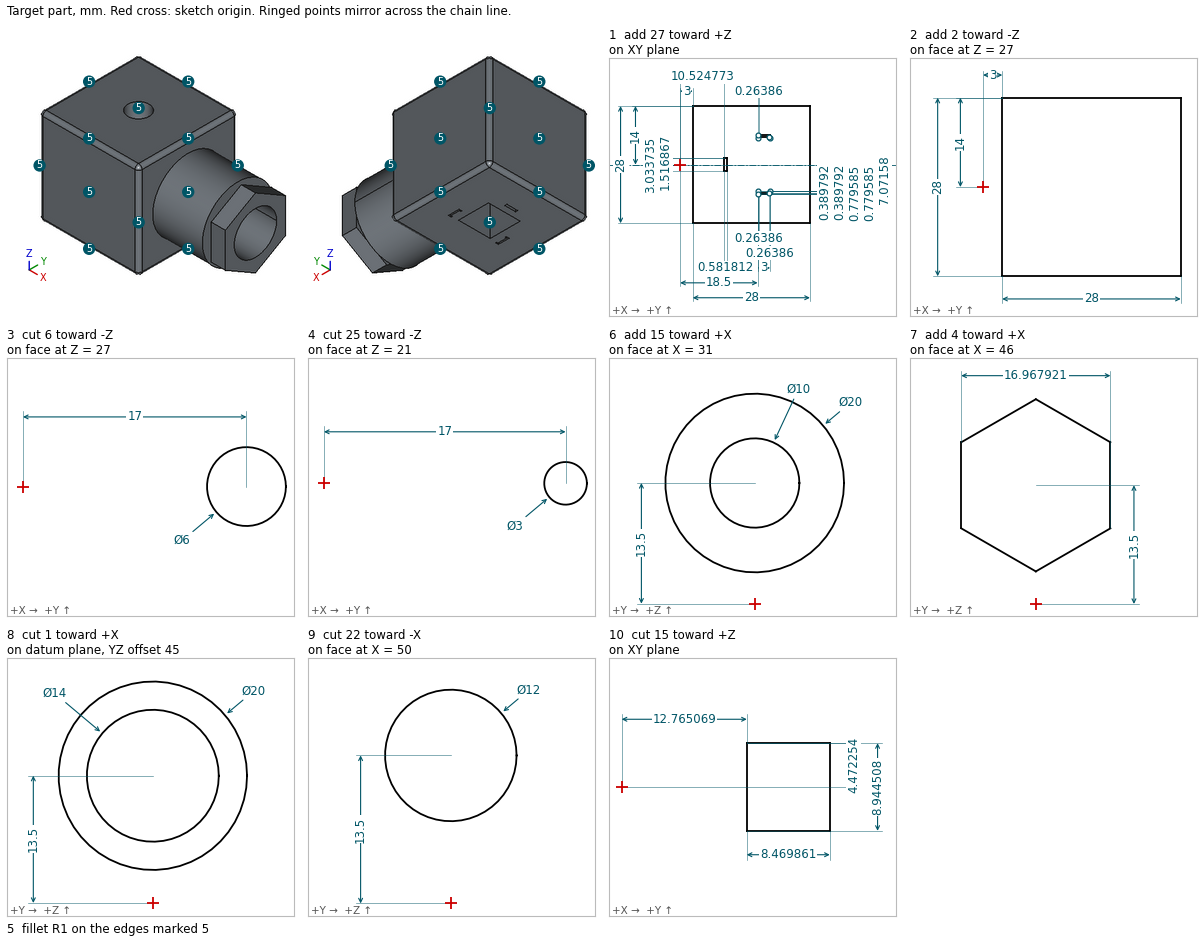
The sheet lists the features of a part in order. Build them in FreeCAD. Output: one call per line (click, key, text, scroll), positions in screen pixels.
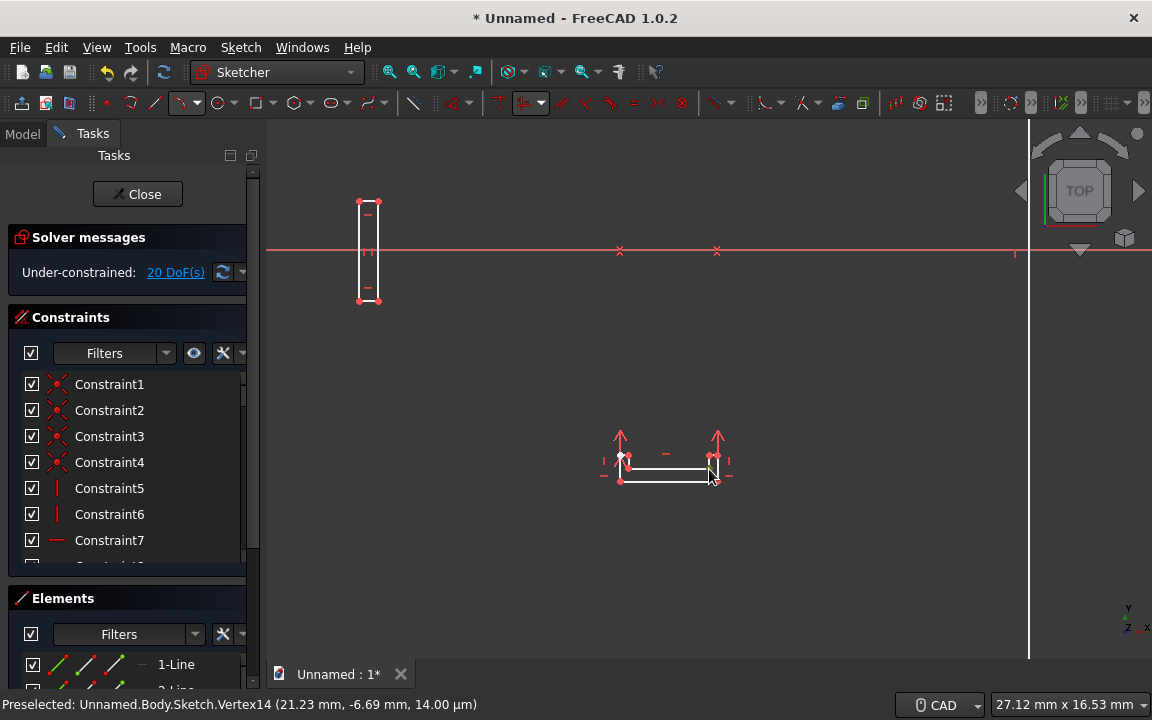
scroll(709, 470, down, 5)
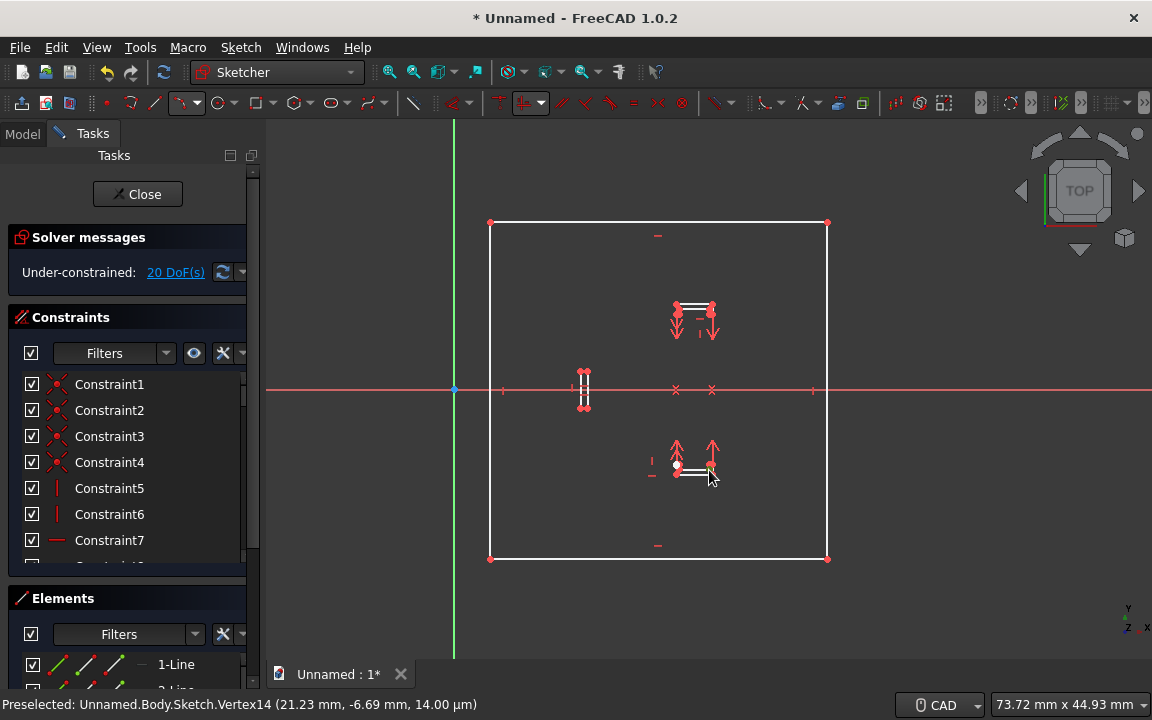
scroll(709, 309, up, 5)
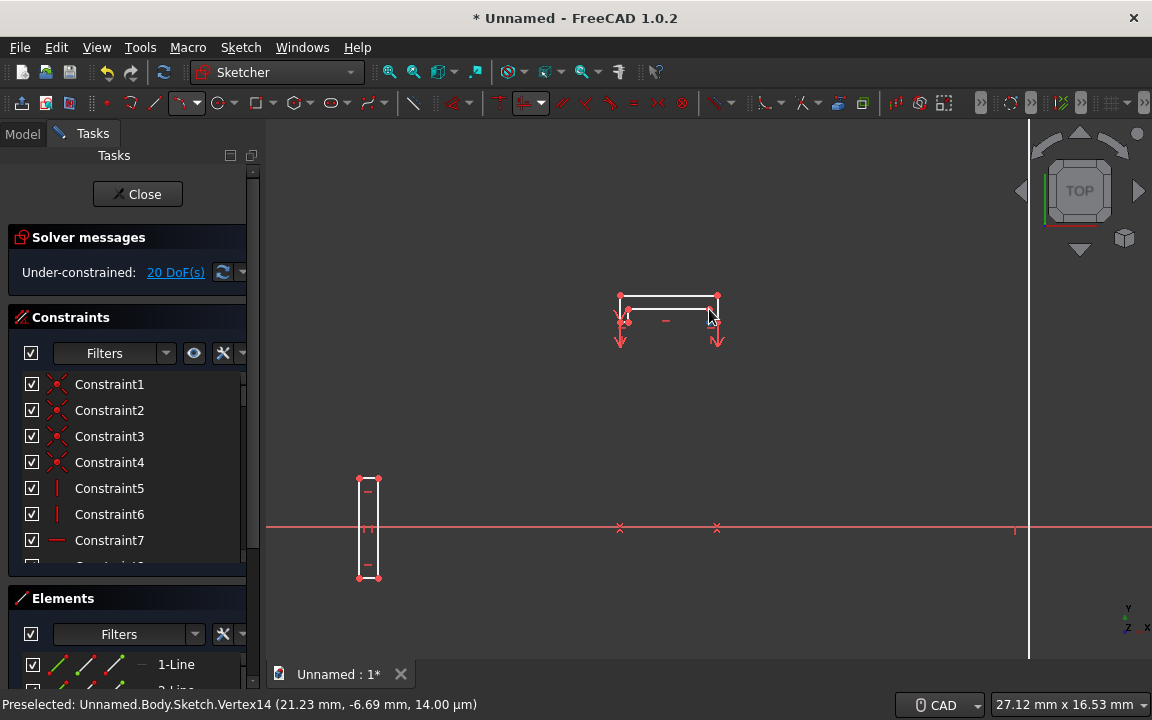
click(709, 309)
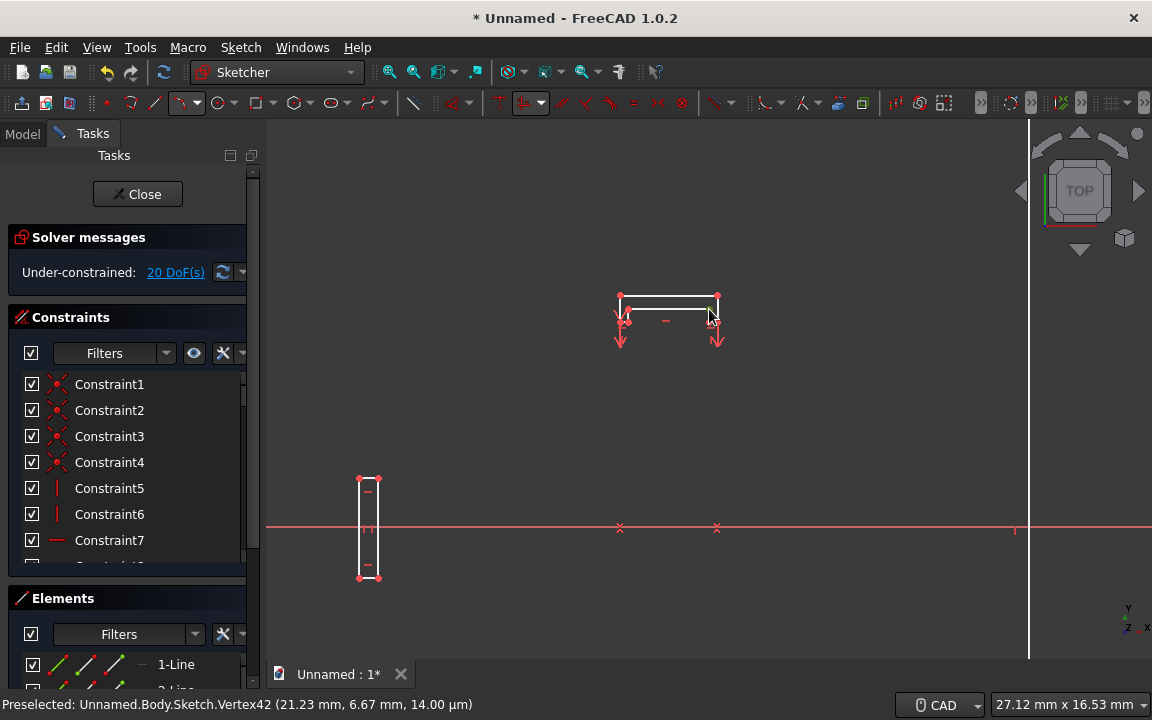
click(442, 527)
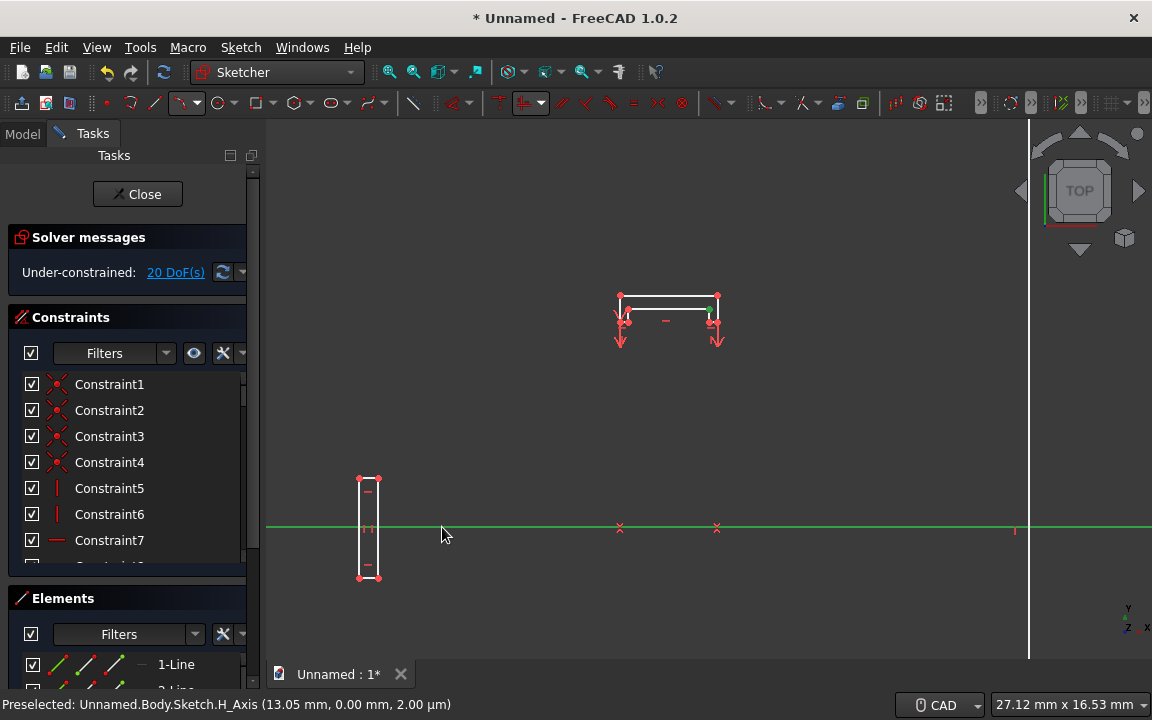
click(658, 104)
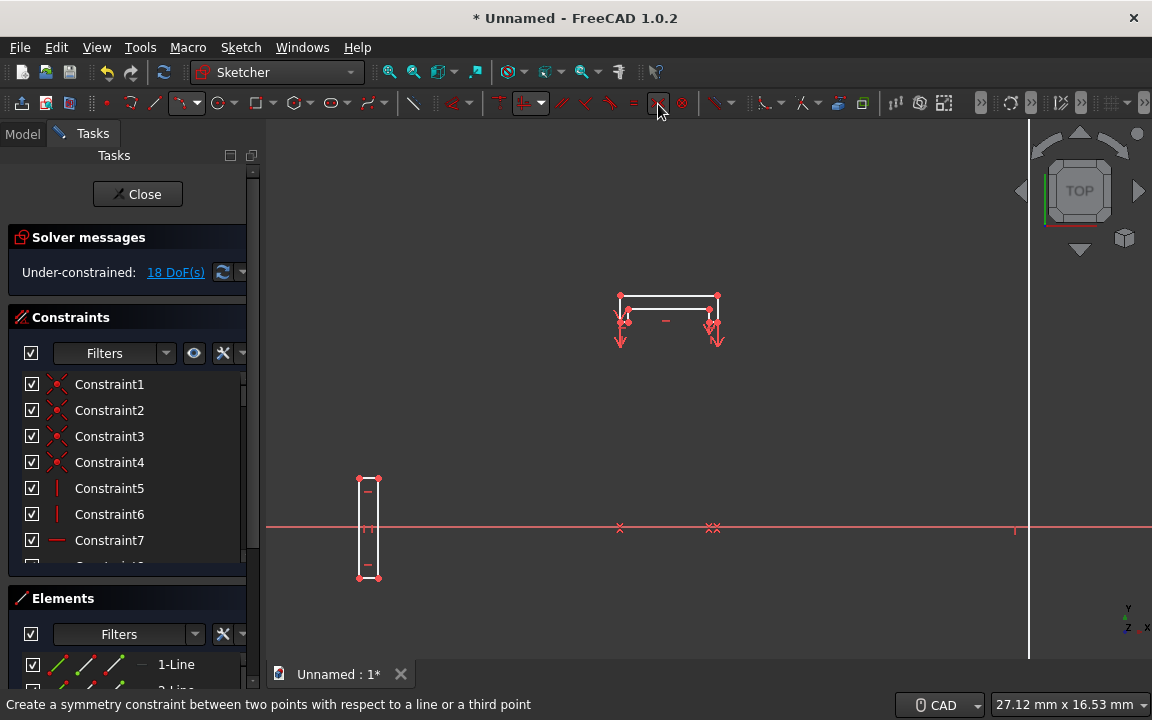
click(452, 104)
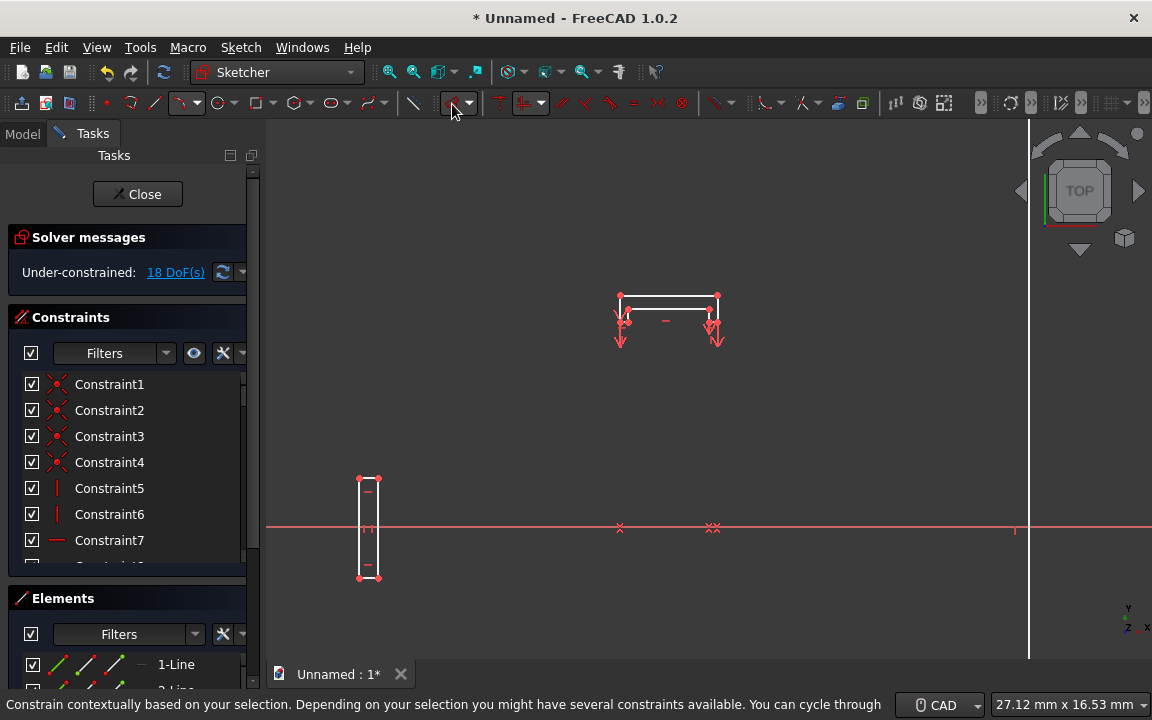
scroll(709, 309, down, 5)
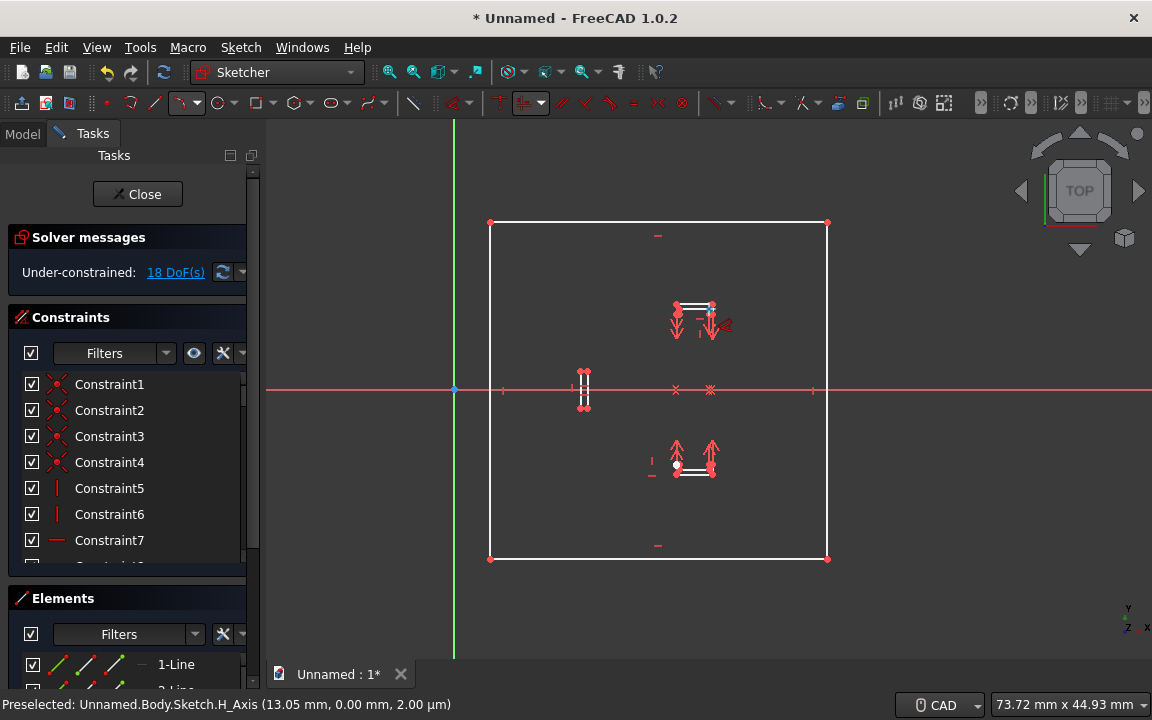
scroll(702, 475, up, 6)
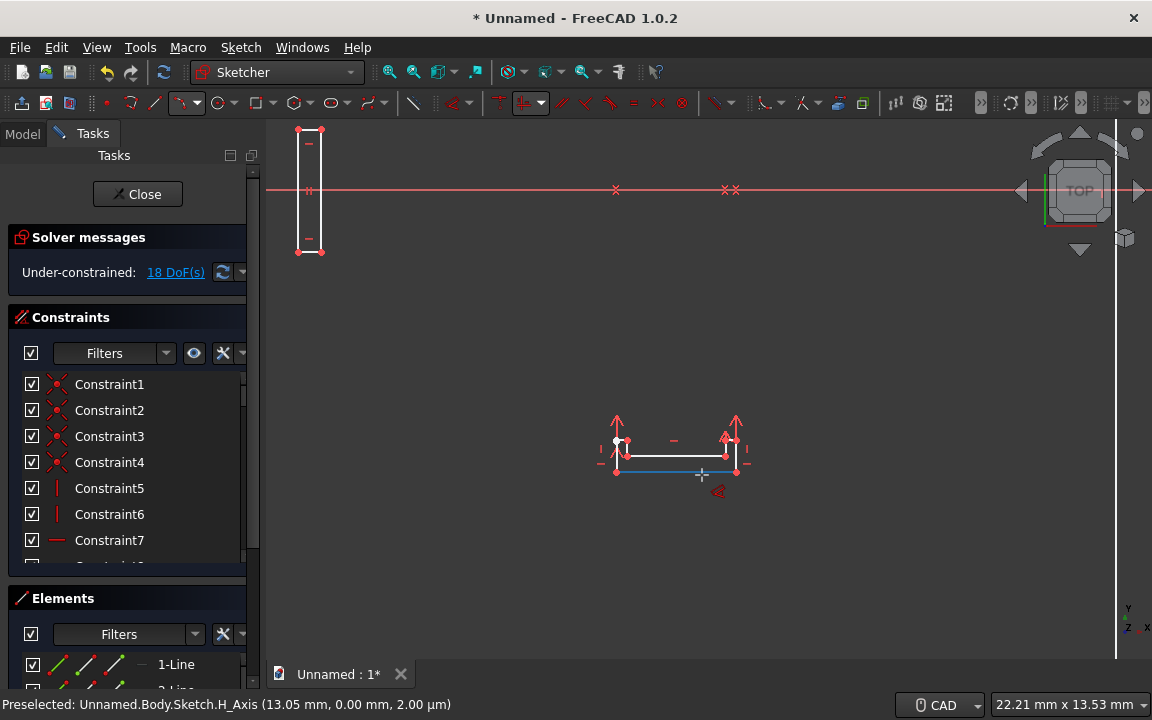
click(700, 472)
click(676, 506)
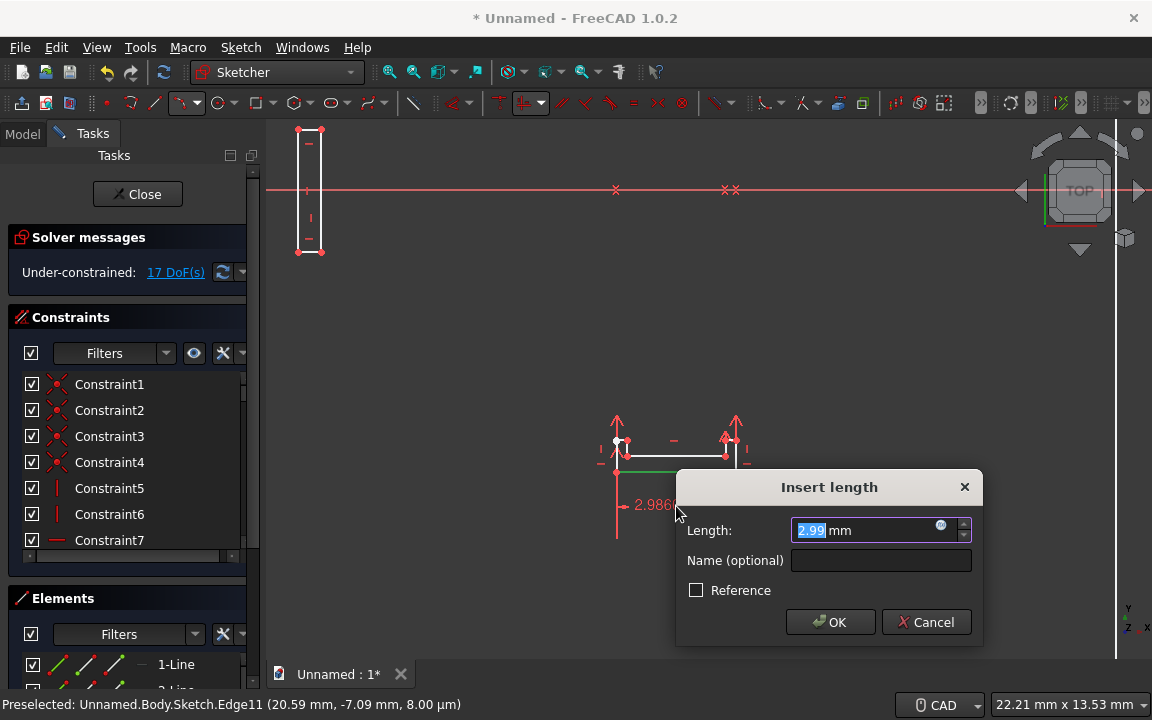
text(3)
key(Return)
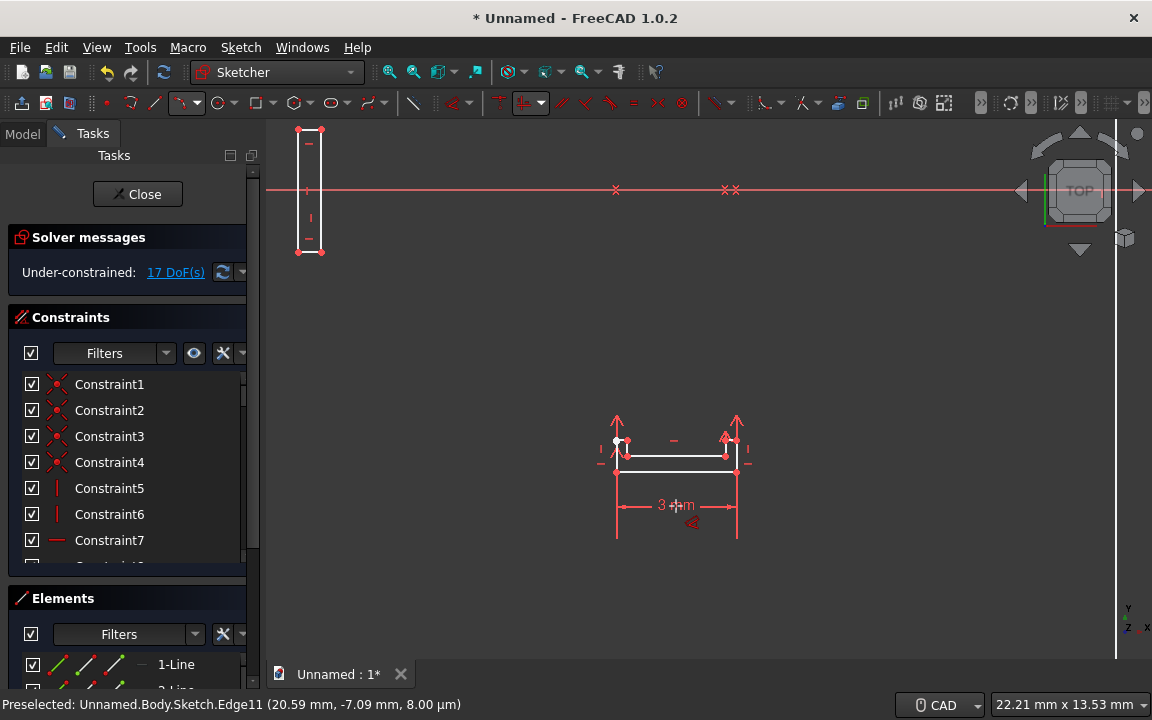
scroll(702, 475, down, 6)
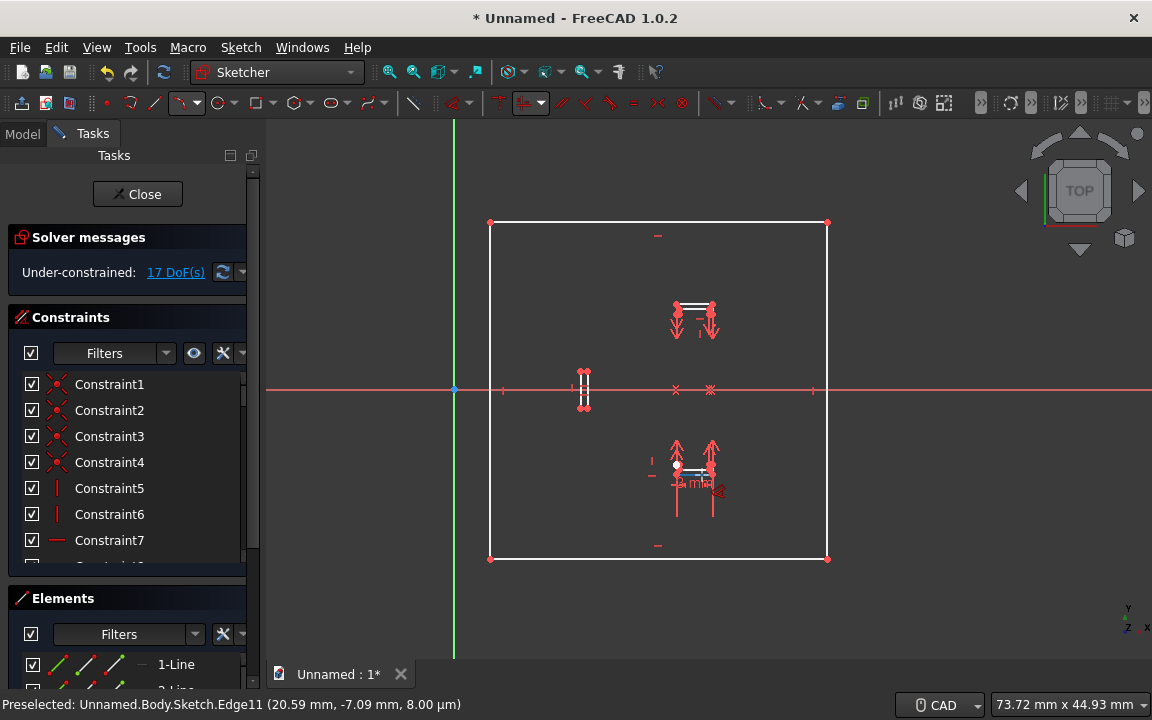
click(490, 323)
click(524, 313)